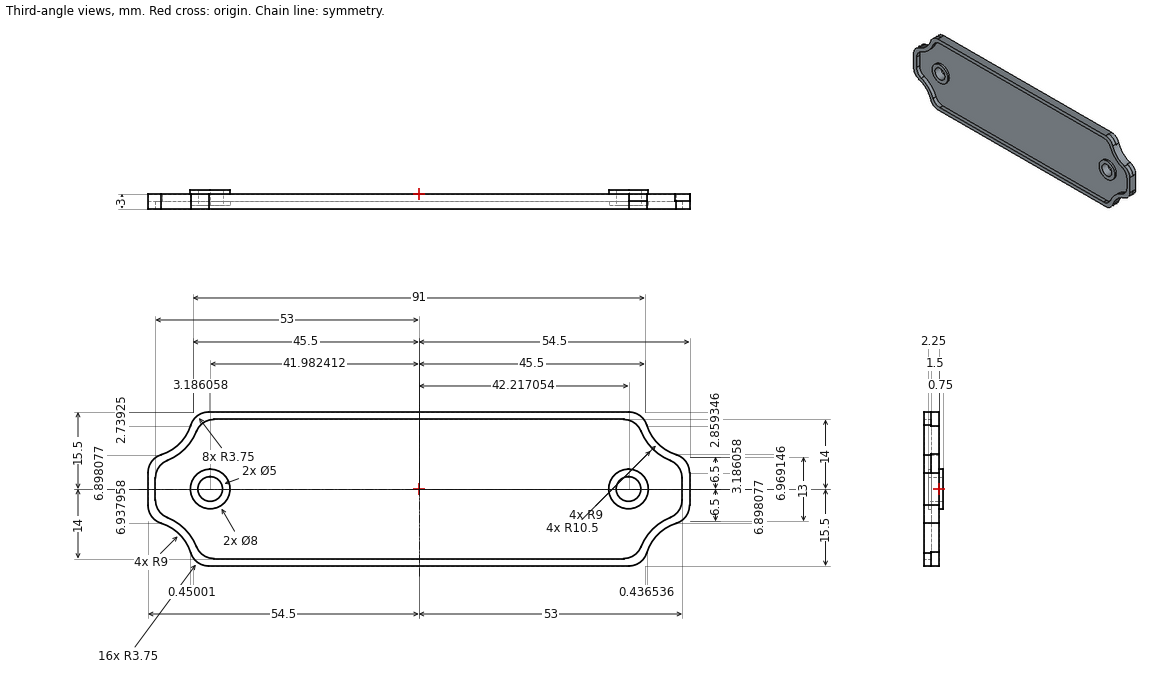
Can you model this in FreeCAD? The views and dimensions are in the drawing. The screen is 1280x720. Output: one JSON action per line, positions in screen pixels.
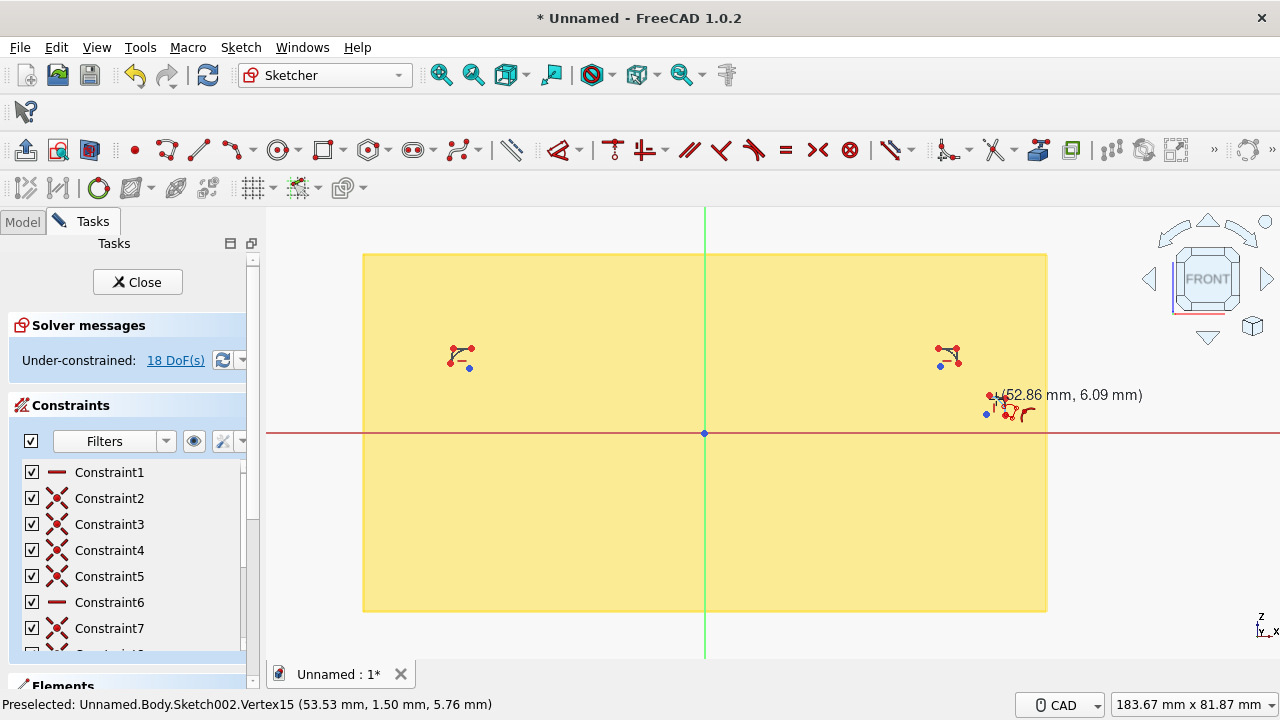
{"action": "left_click", "coordinate": [991, 471]}
{"action": "left_click", "coordinate": [1006, 469]}
{"action": "left_click", "coordinate": [1006, 451]}
{"action": "right_click", "coordinate": [1006, 451]}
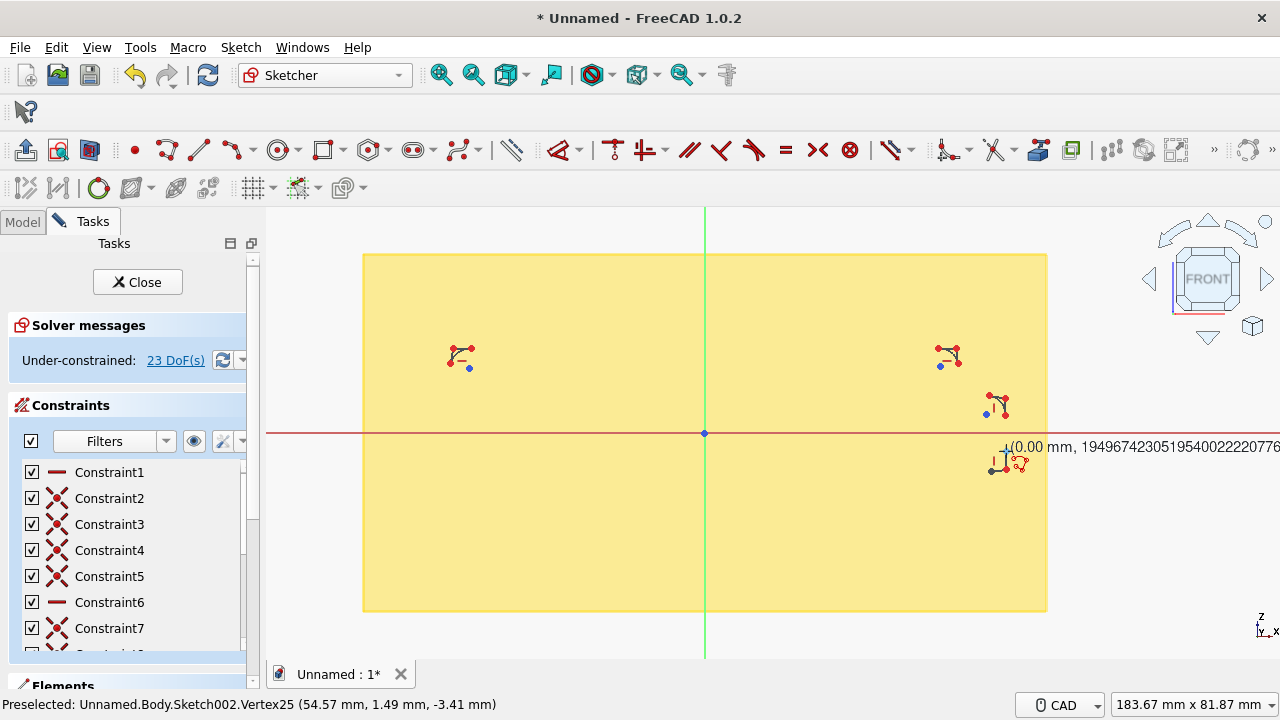
{"action": "left_click", "coordinate": [232, 150]}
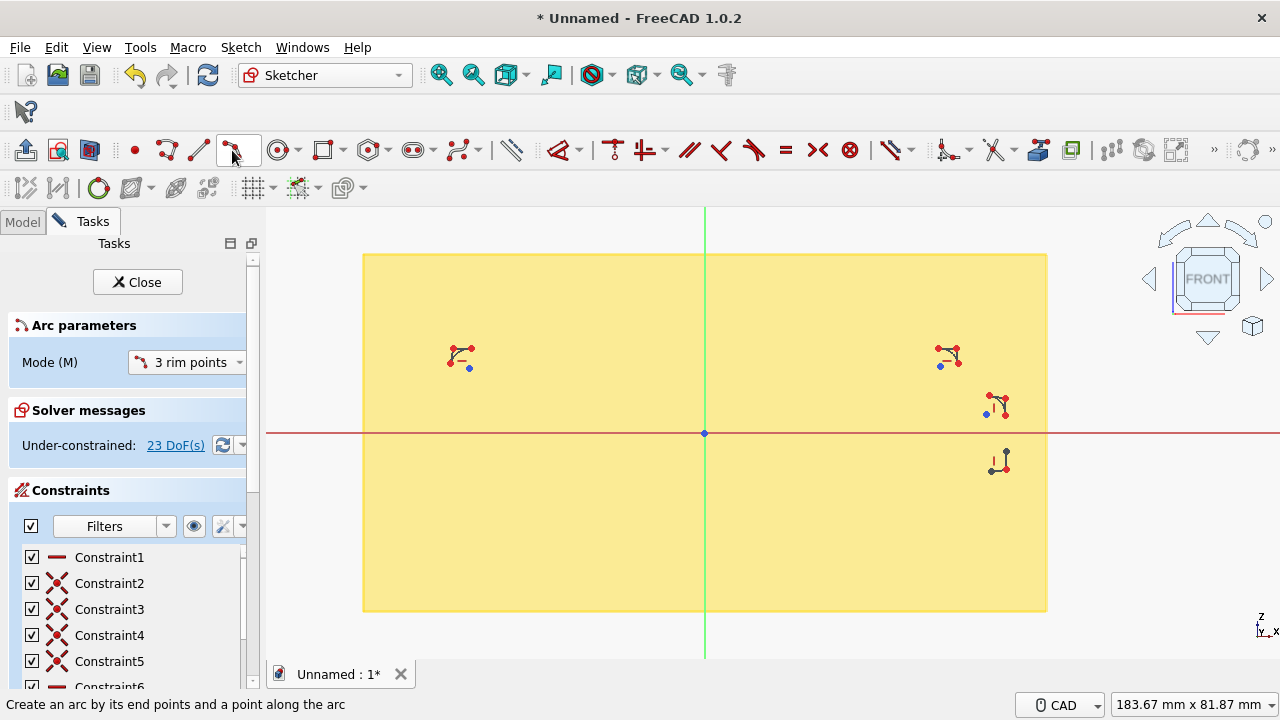
{"action": "scroll", "coordinate": [1006, 451], "scroll_direction": "up", "scroll_amount": 3}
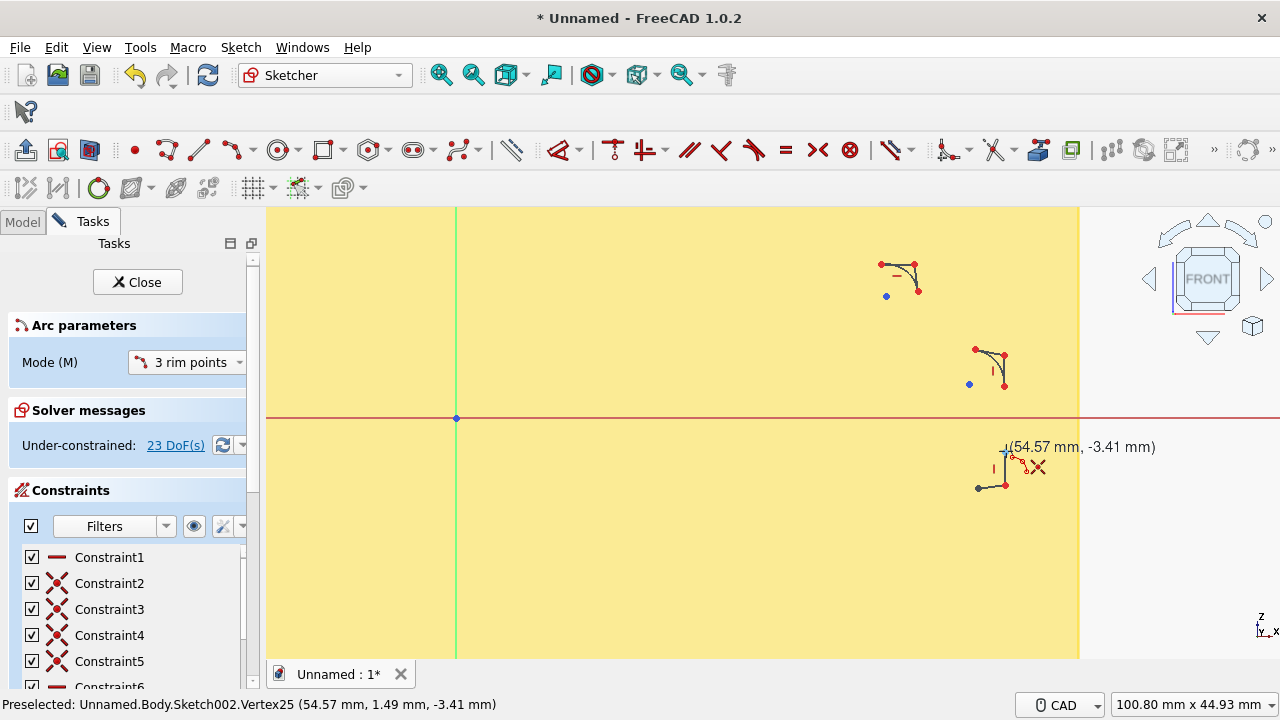
{"action": "left_click", "coordinate": [1005, 452]}
{"action": "left_click", "coordinate": [978, 489]}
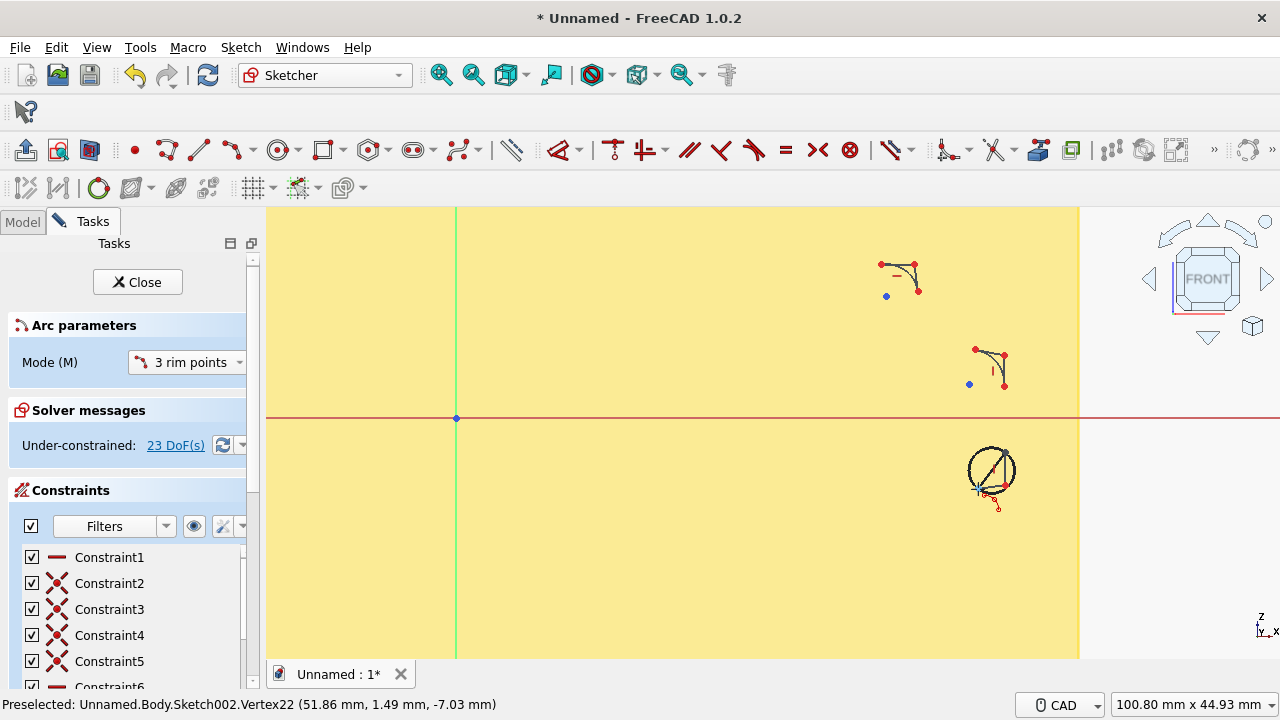
{"action": "scroll", "coordinate": [997, 474], "scroll_direction": "up", "scroll_amount": 4}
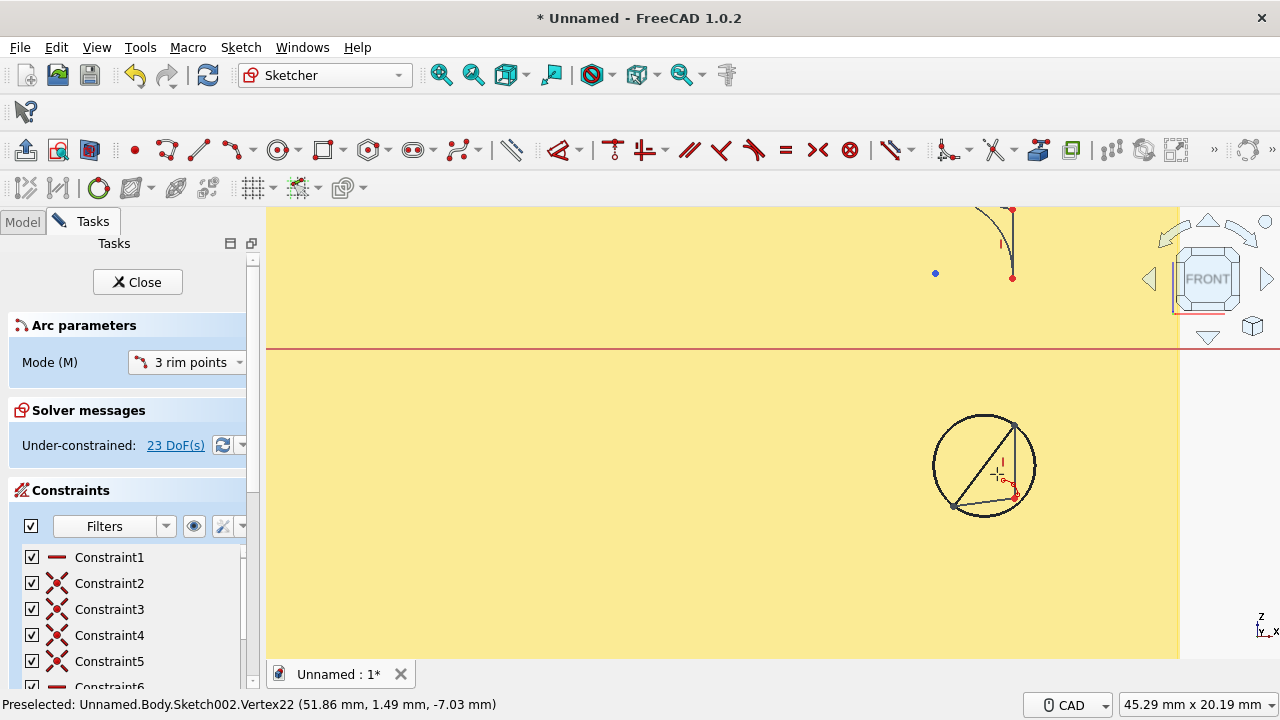
{"action": "left_click", "coordinate": [997, 473]}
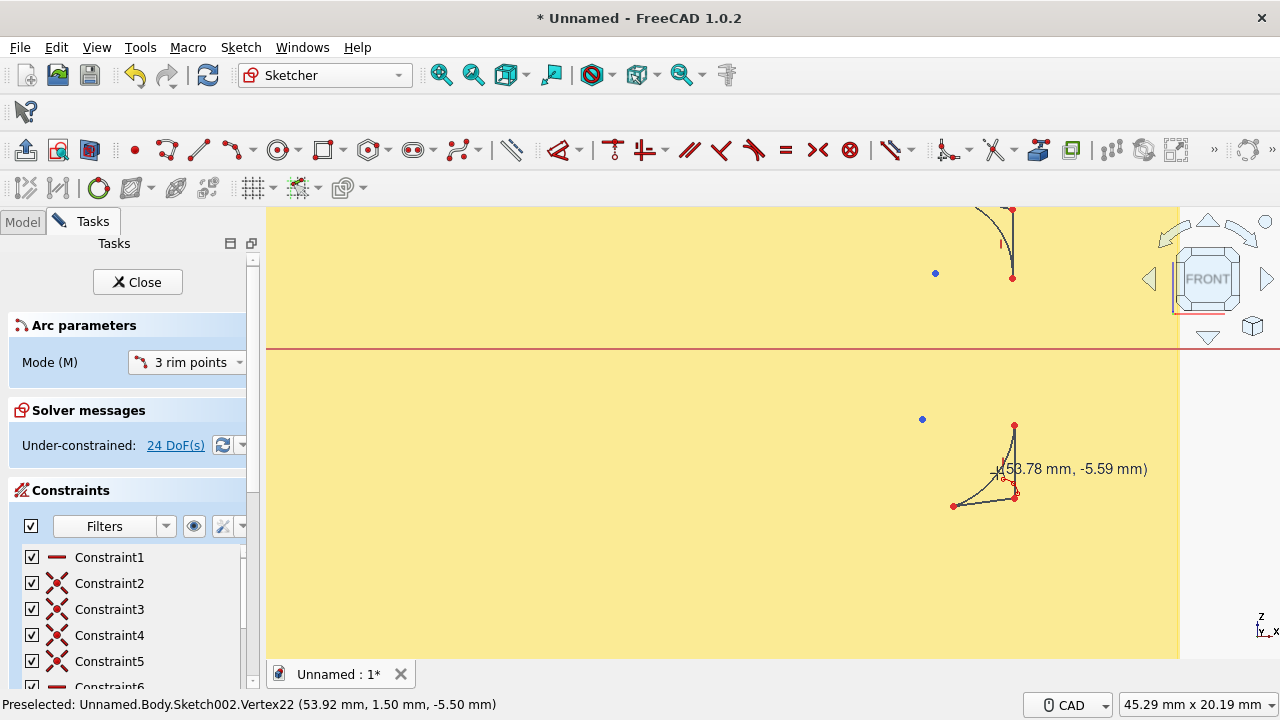
{"action": "left_click", "coordinate": [168, 150]}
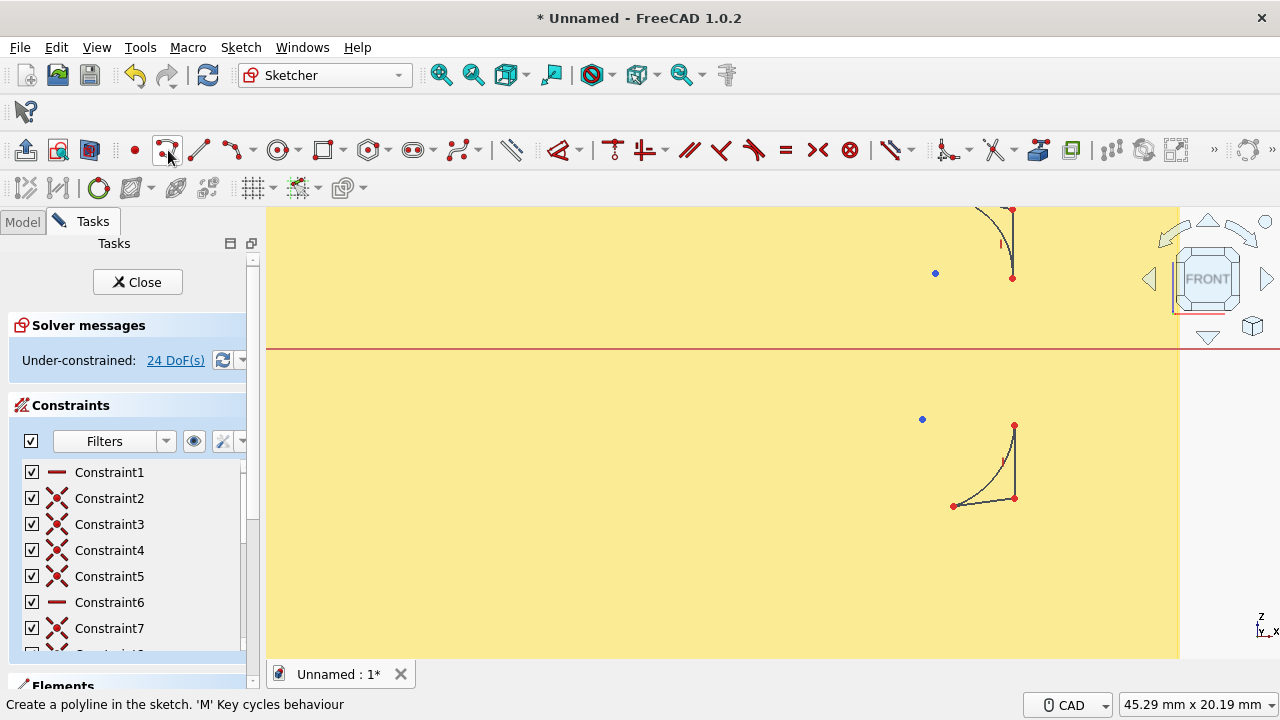
{"action": "scroll", "coordinate": [1003, 461], "scroll_direction": "down", "scroll_amount": 7}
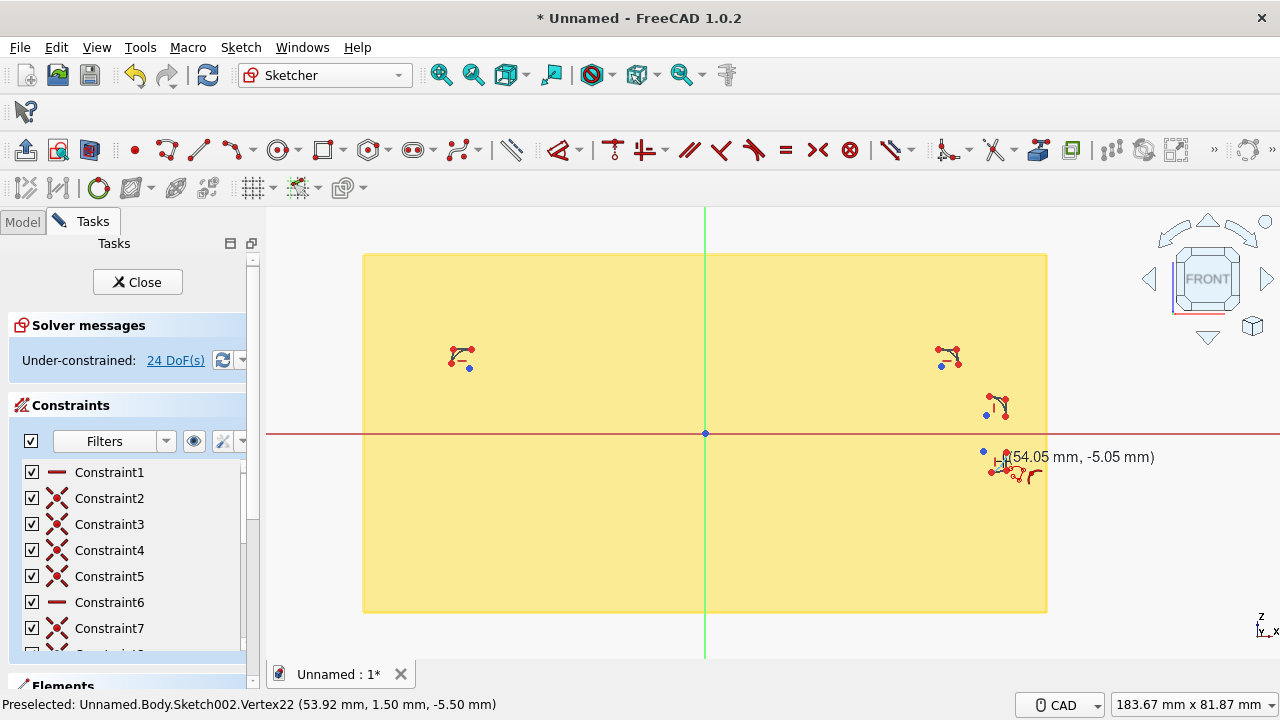
{"action": "left_click", "coordinate": [939, 519]}
{"action": "left_click", "coordinate": [956, 519]}
{"action": "left_click", "coordinate": [959, 504]}
{"action": "right_click", "coordinate": [959, 504]}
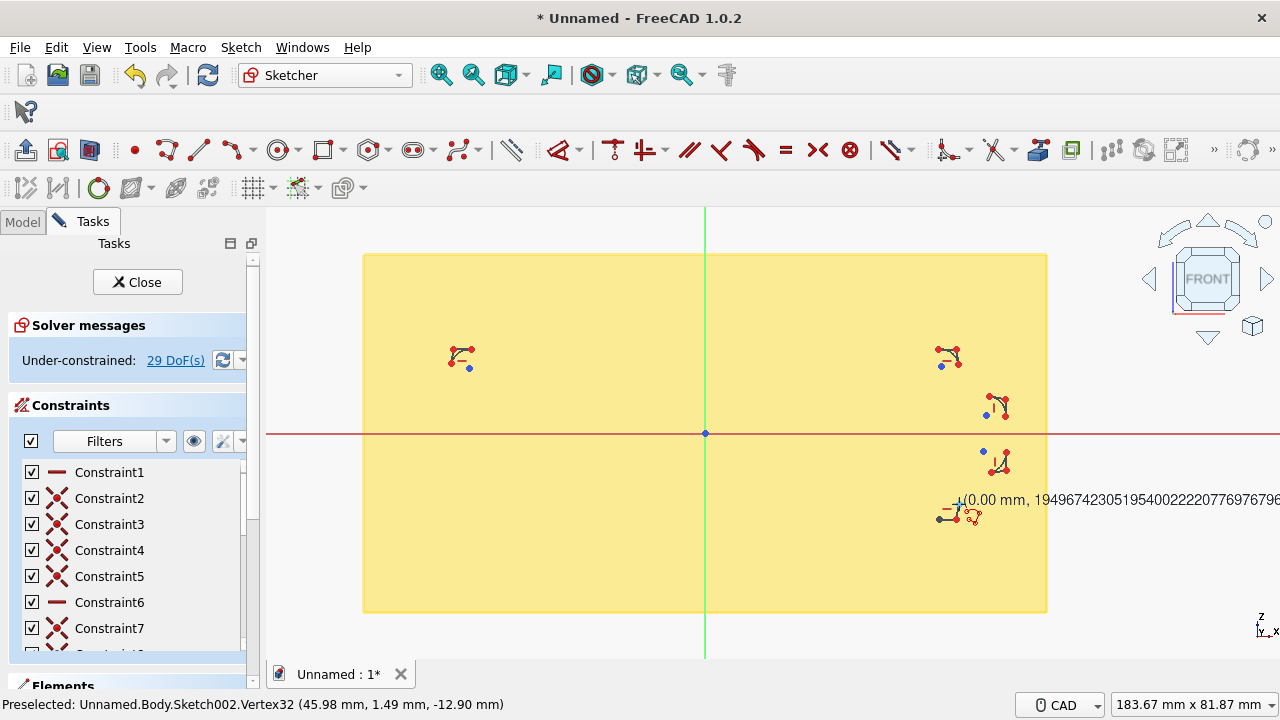
{"action": "left_click", "coordinate": [232, 150]}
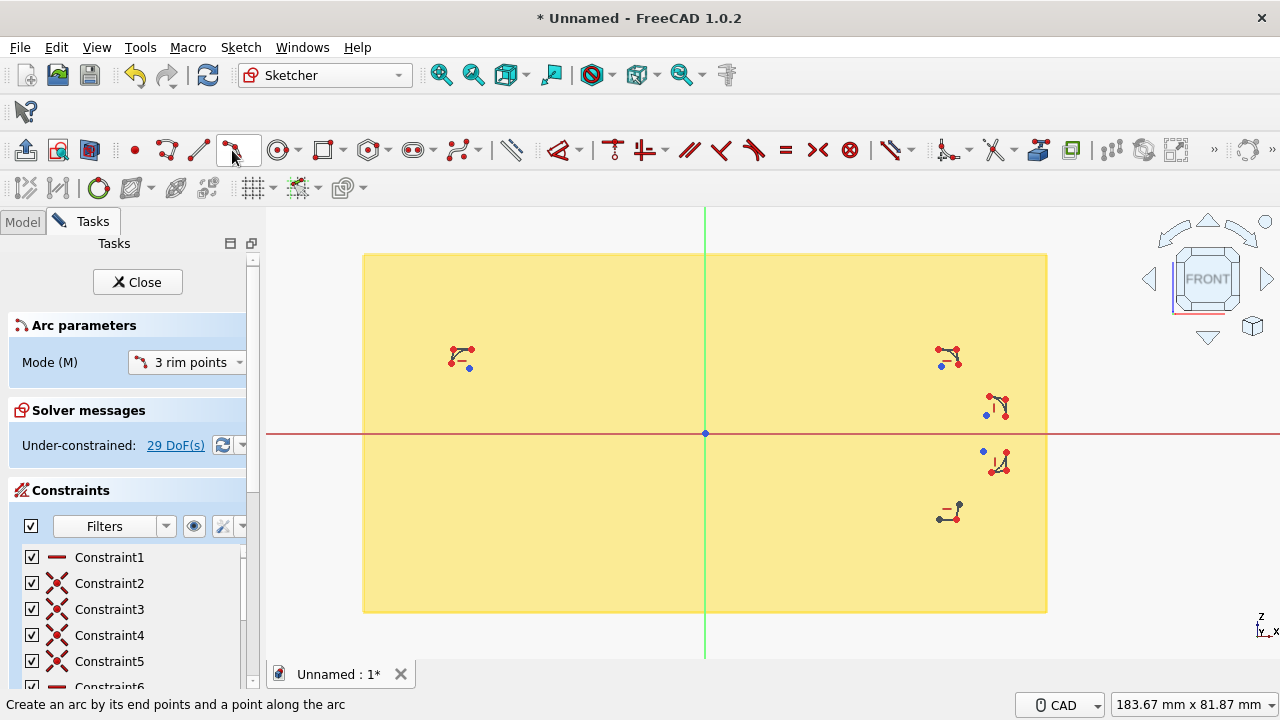
{"action": "scroll", "coordinate": [959, 504], "scroll_direction": "up", "scroll_amount": 4}